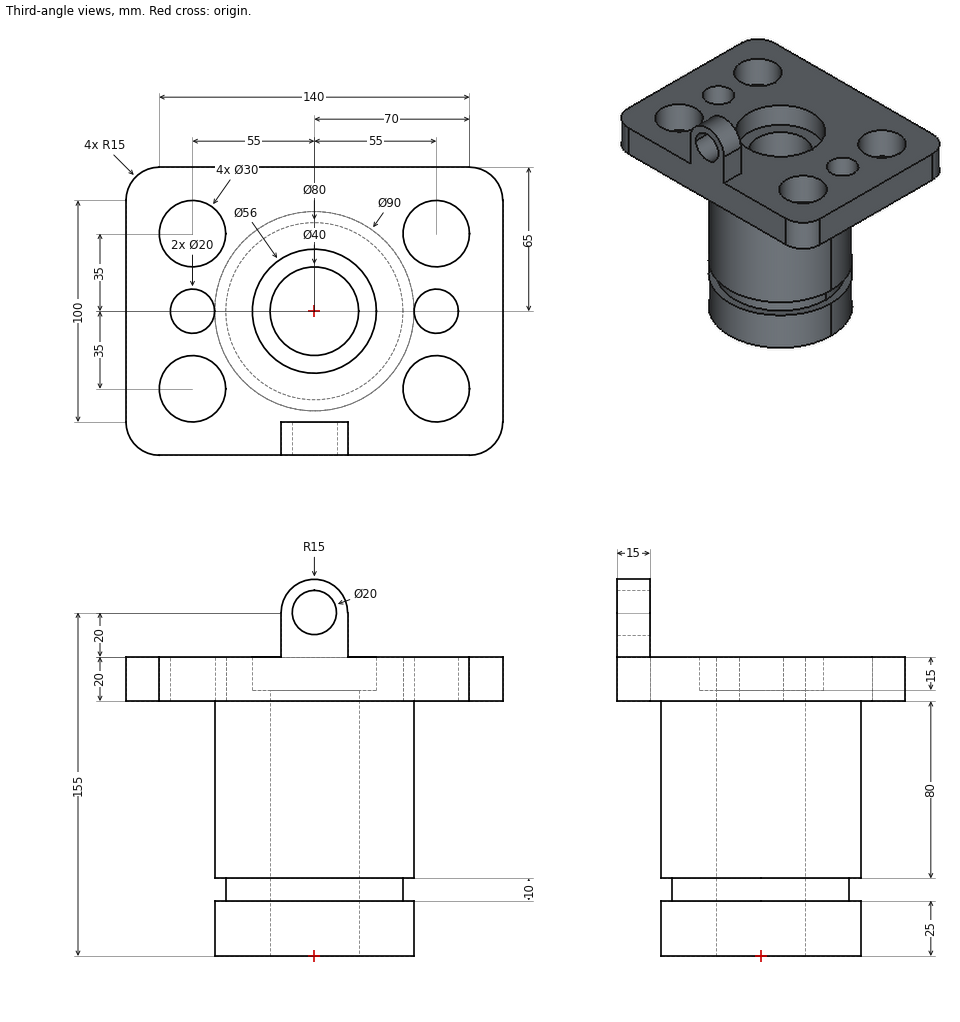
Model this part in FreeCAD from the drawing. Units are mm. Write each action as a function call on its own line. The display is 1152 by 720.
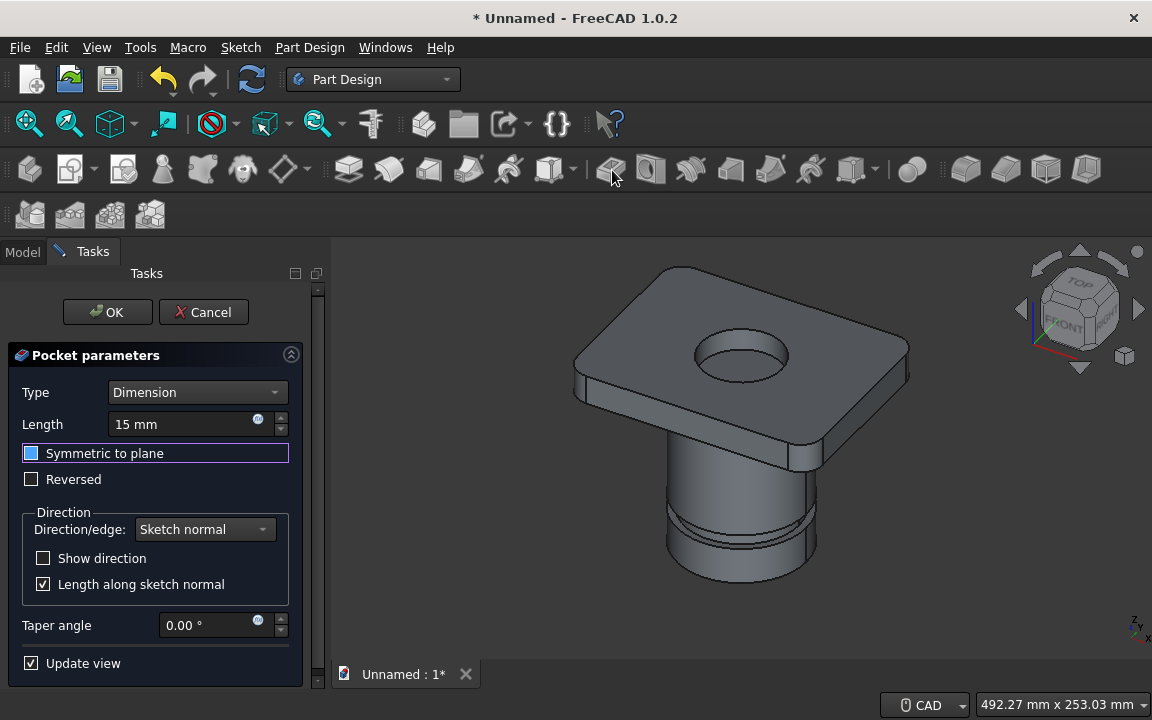
click(108, 312)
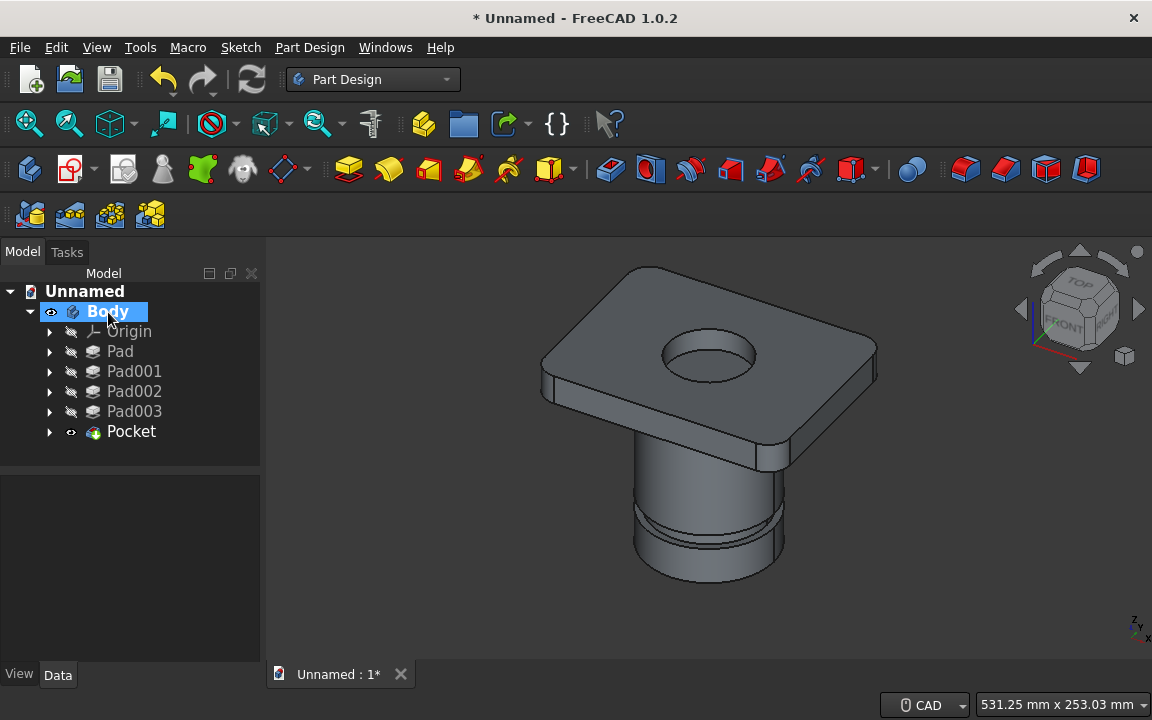
click(716, 369)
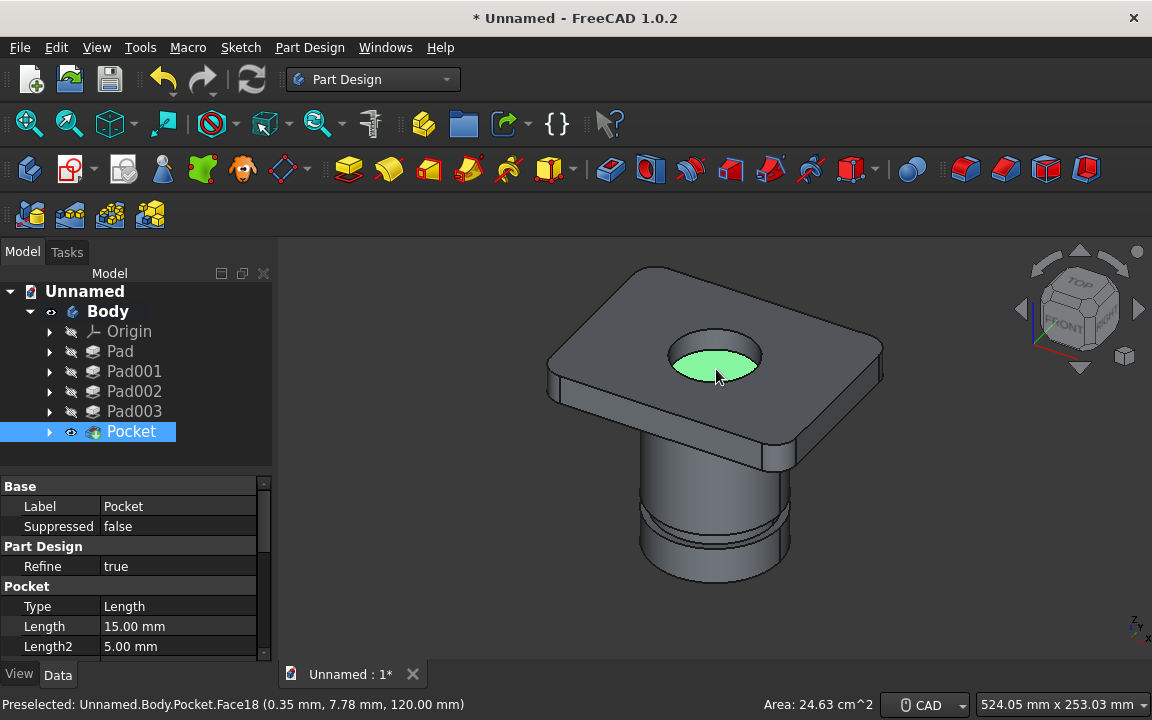
click(70, 170)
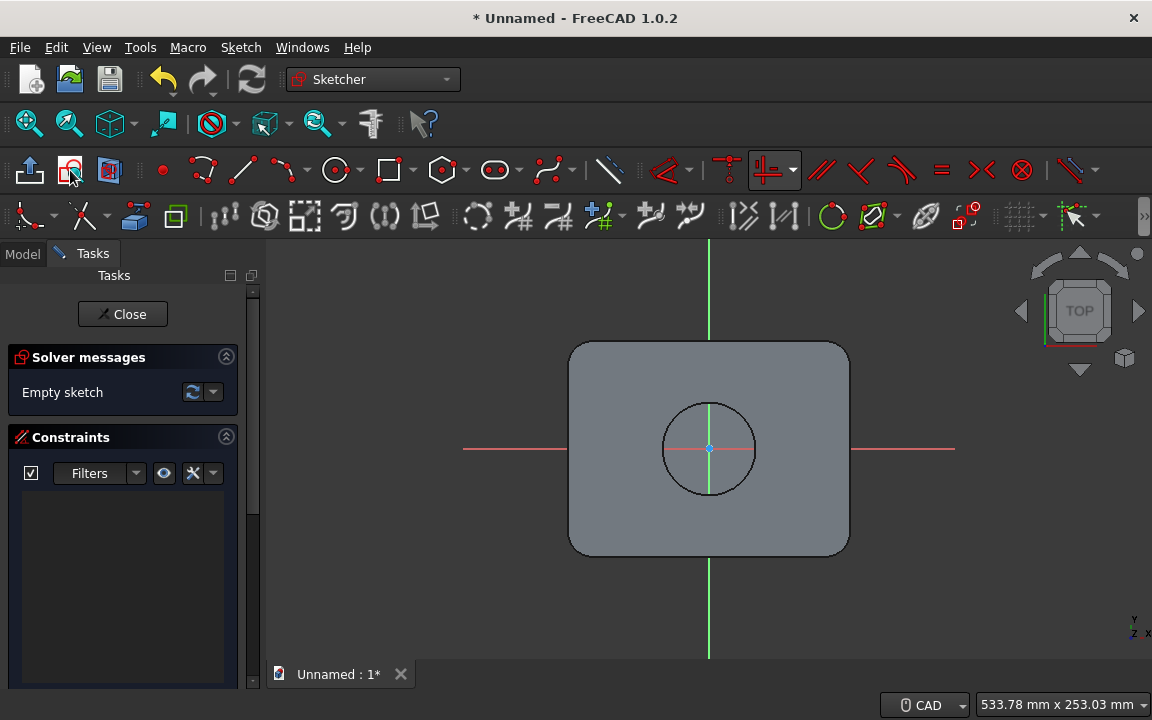
click(110, 170)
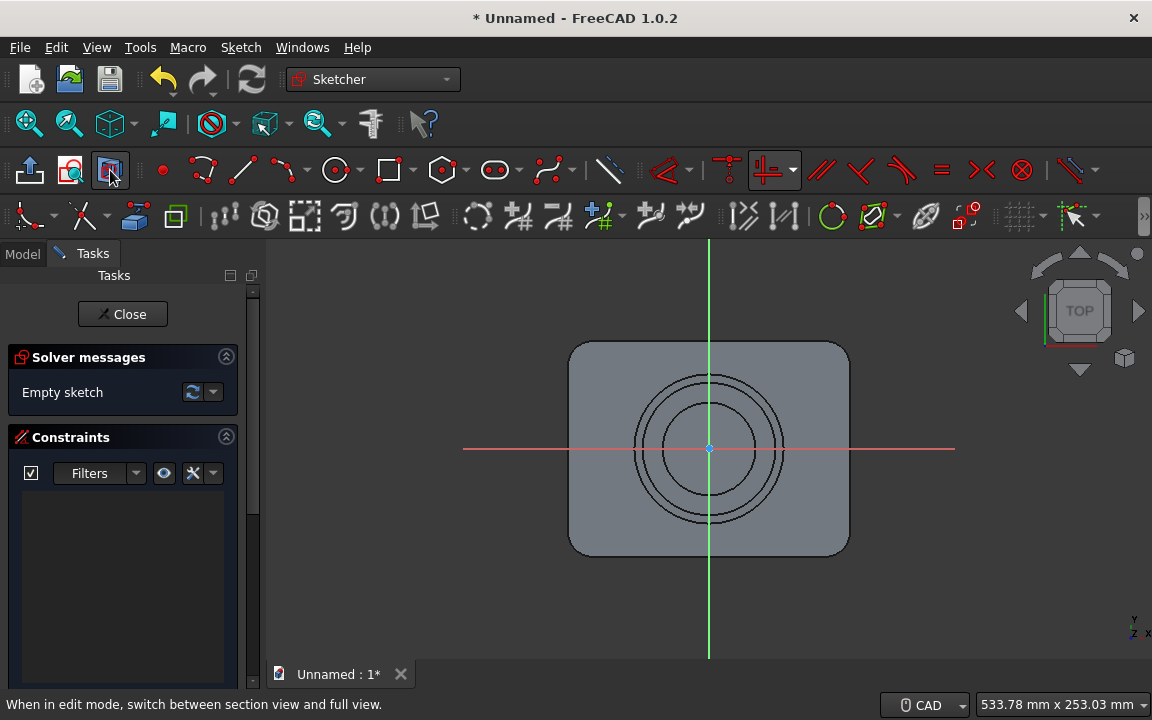
scroll(731, 449, up, 7)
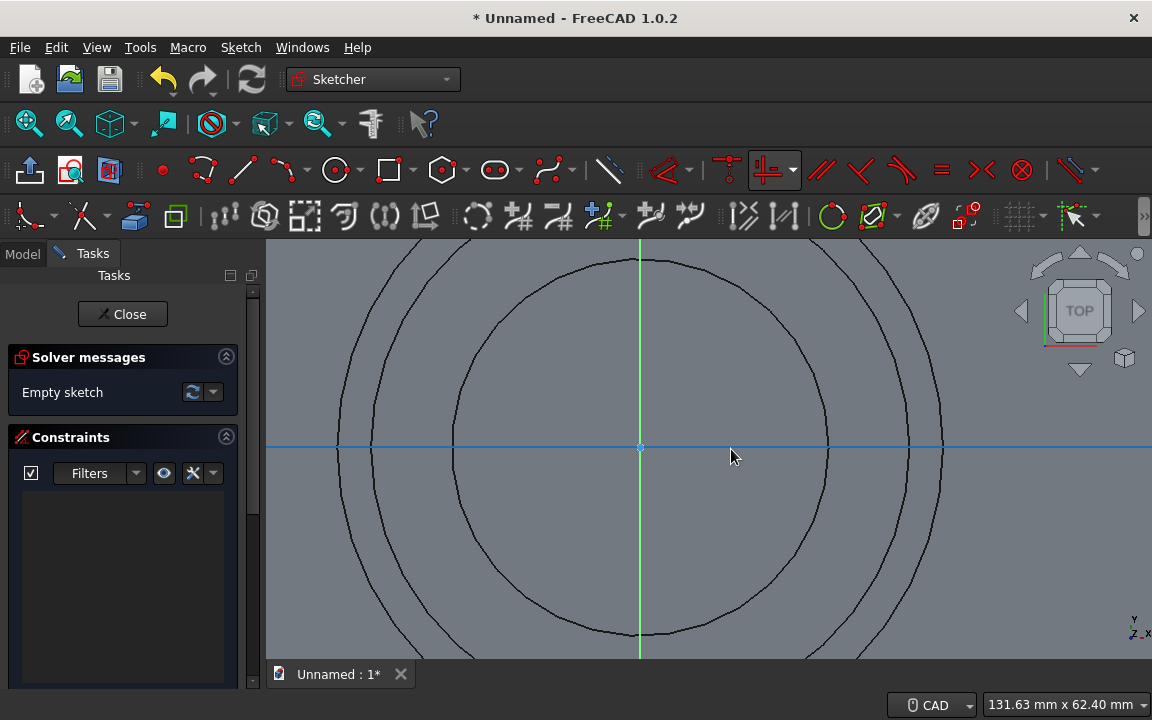
click(336, 170)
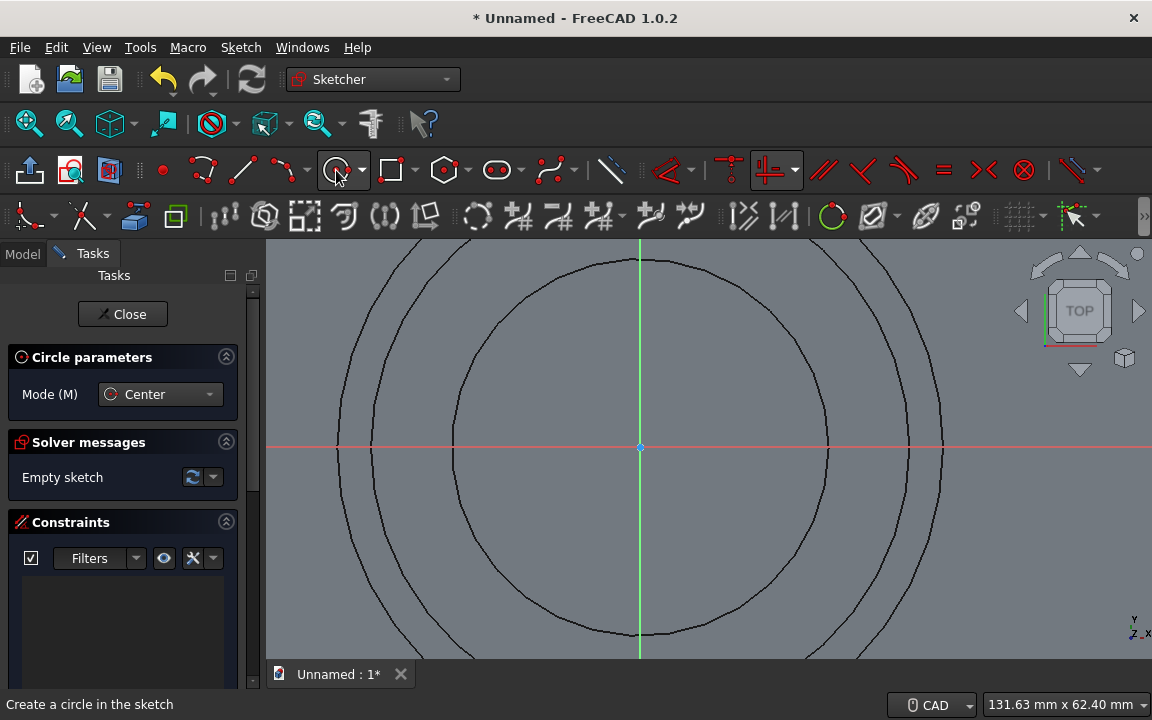
click(640, 447)
click(735, 352)
key(Escape)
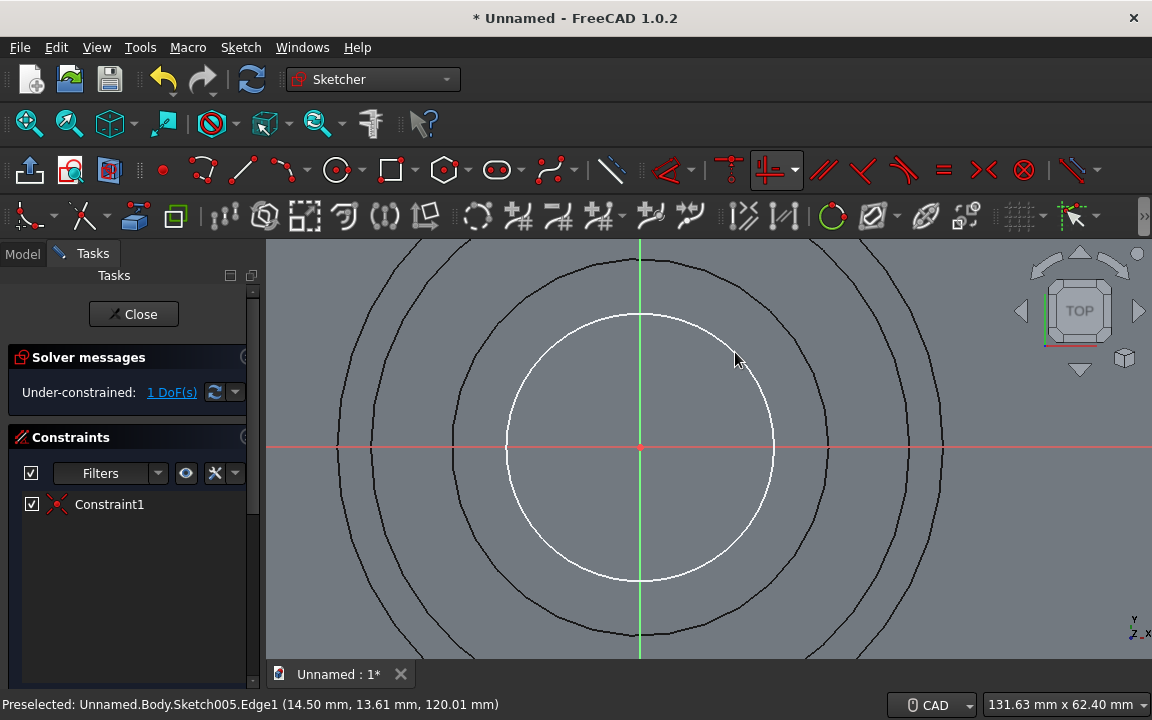
click(666, 170)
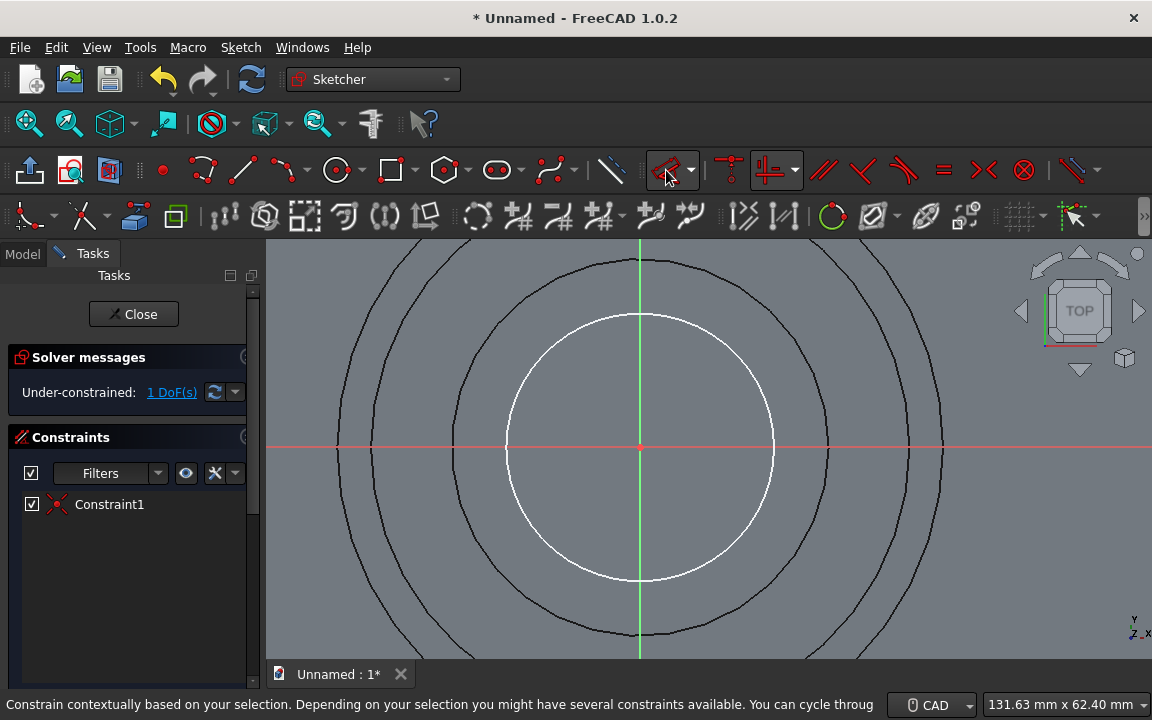
click(735, 353)
click(758, 330)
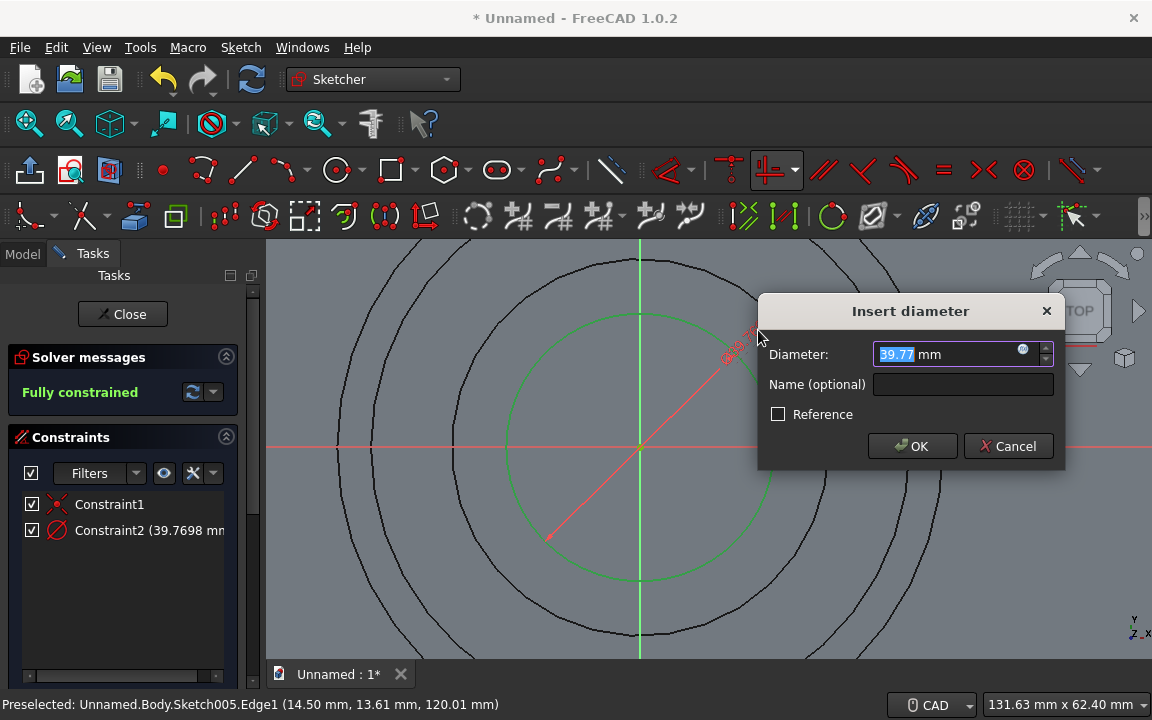
text(40)
key(Return)
key(Escape)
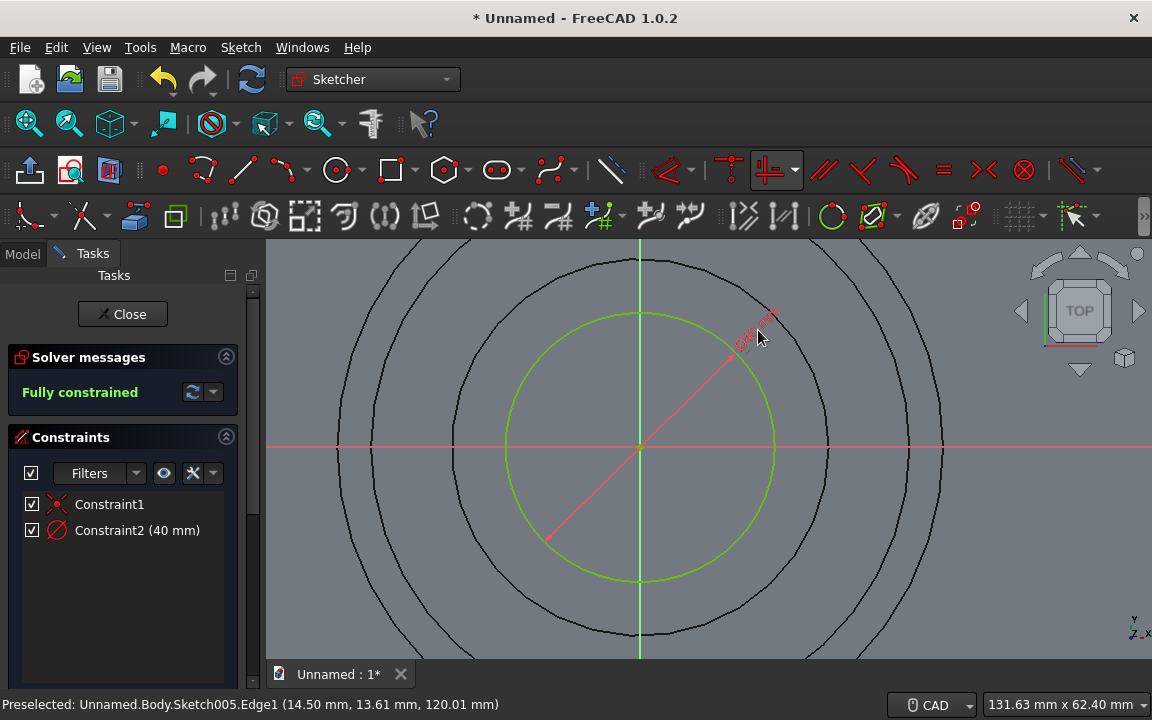
click(123, 314)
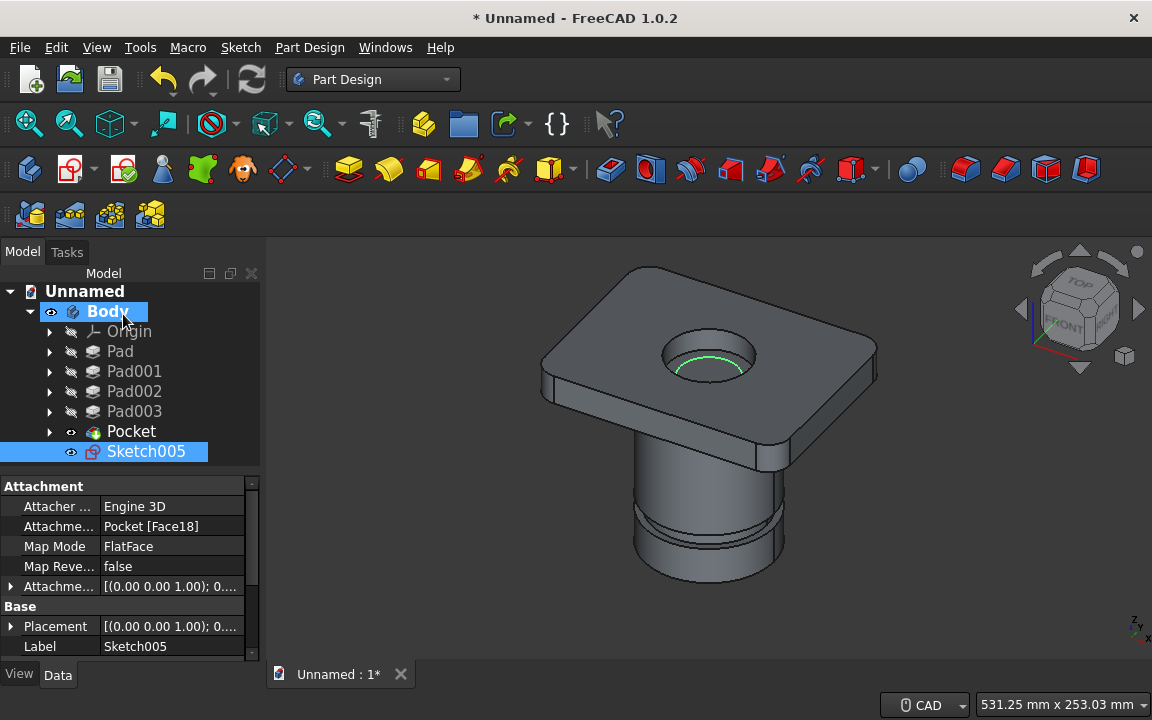
click(612, 170)